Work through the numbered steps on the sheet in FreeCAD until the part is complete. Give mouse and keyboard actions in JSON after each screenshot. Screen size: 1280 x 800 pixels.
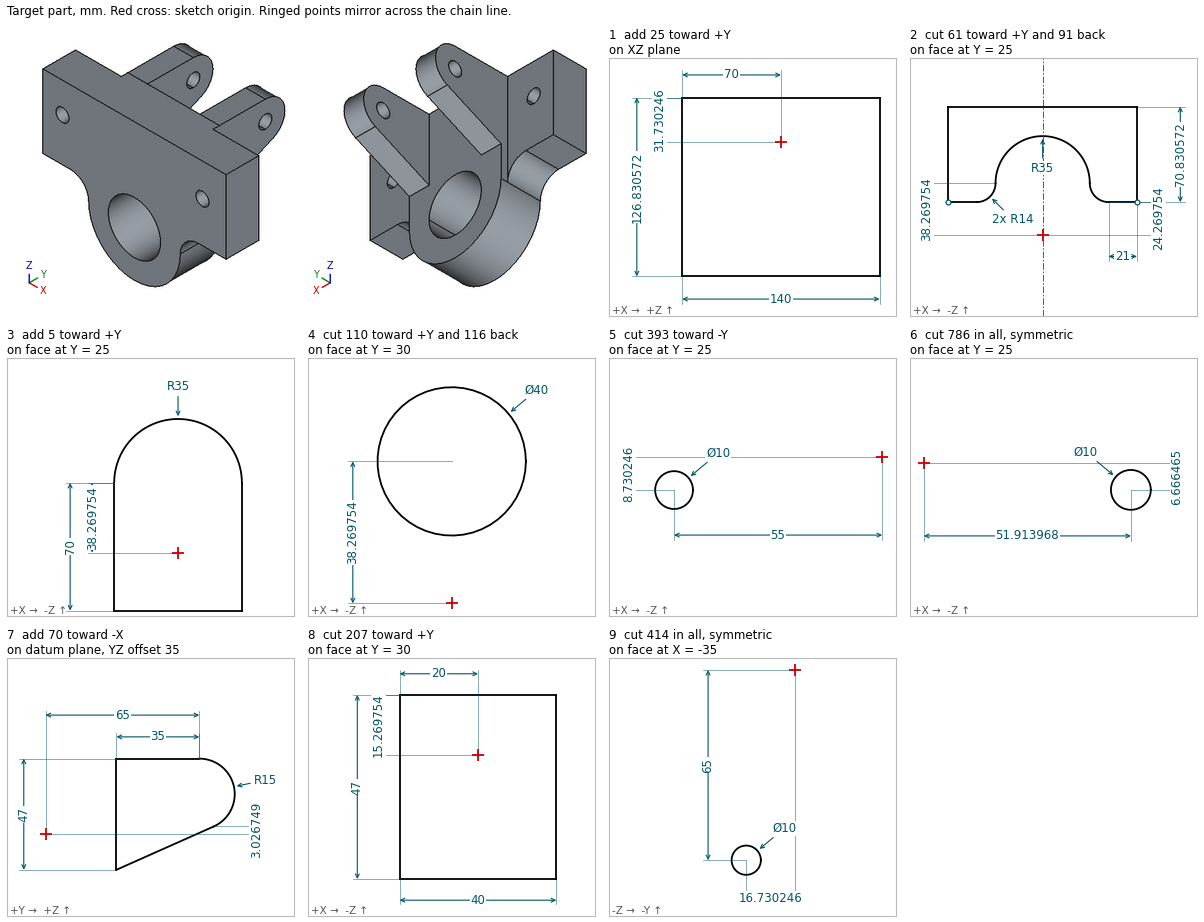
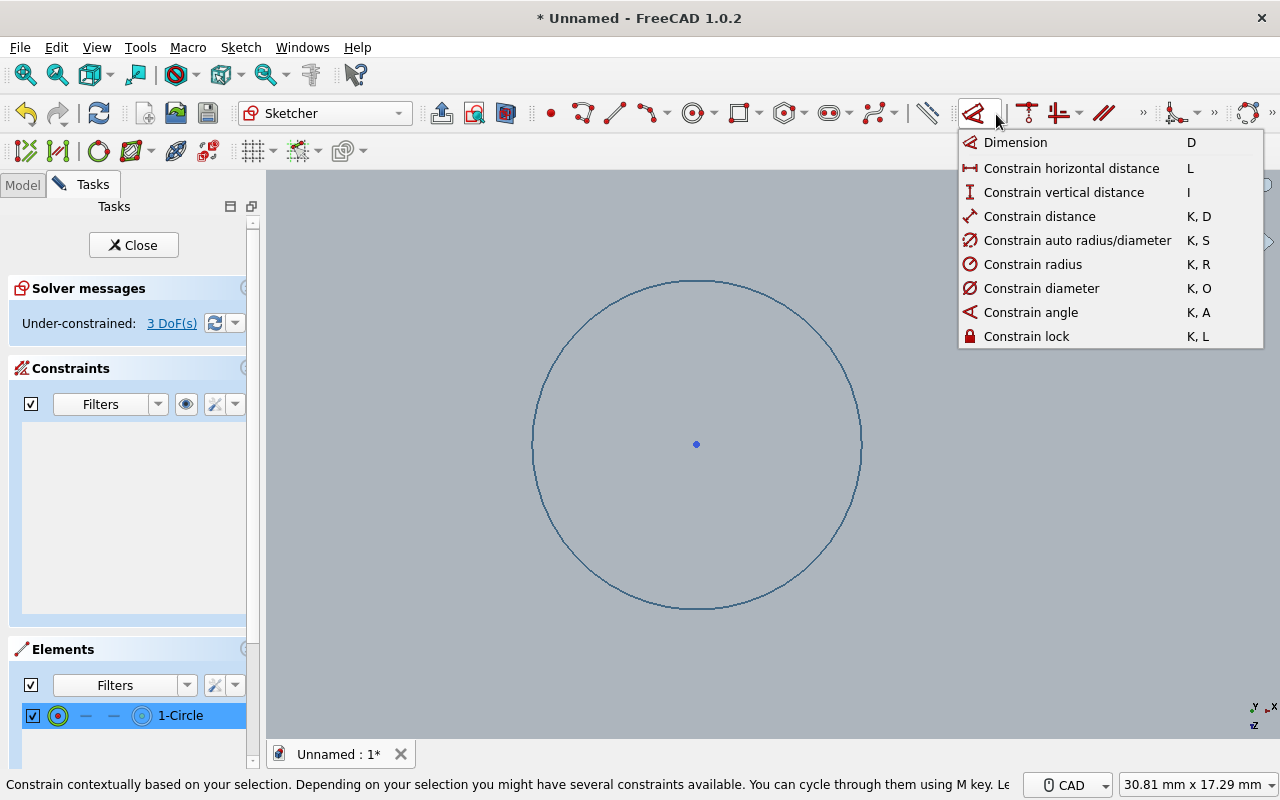
{"action": "left_click", "coordinate": [1111, 288]}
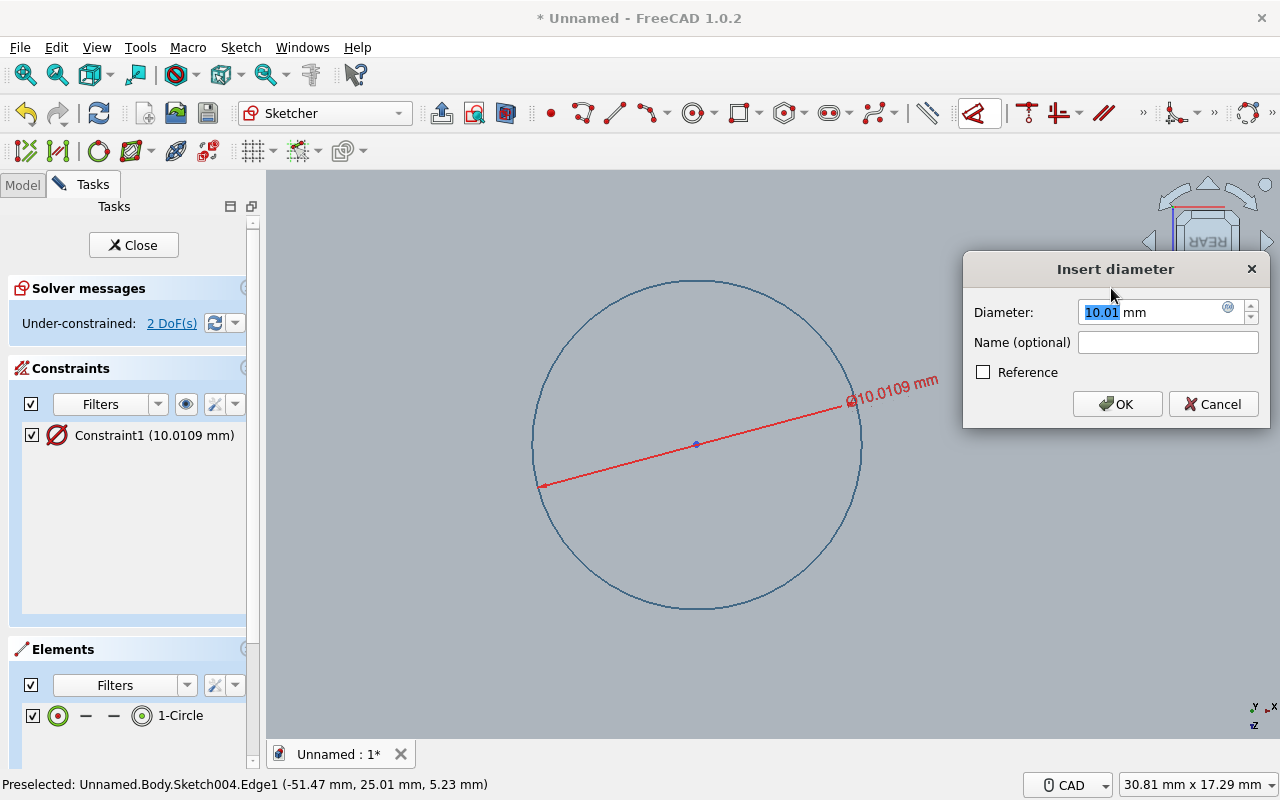
{"action": "type", "text": "10"}
{"action": "key", "text": "Return"}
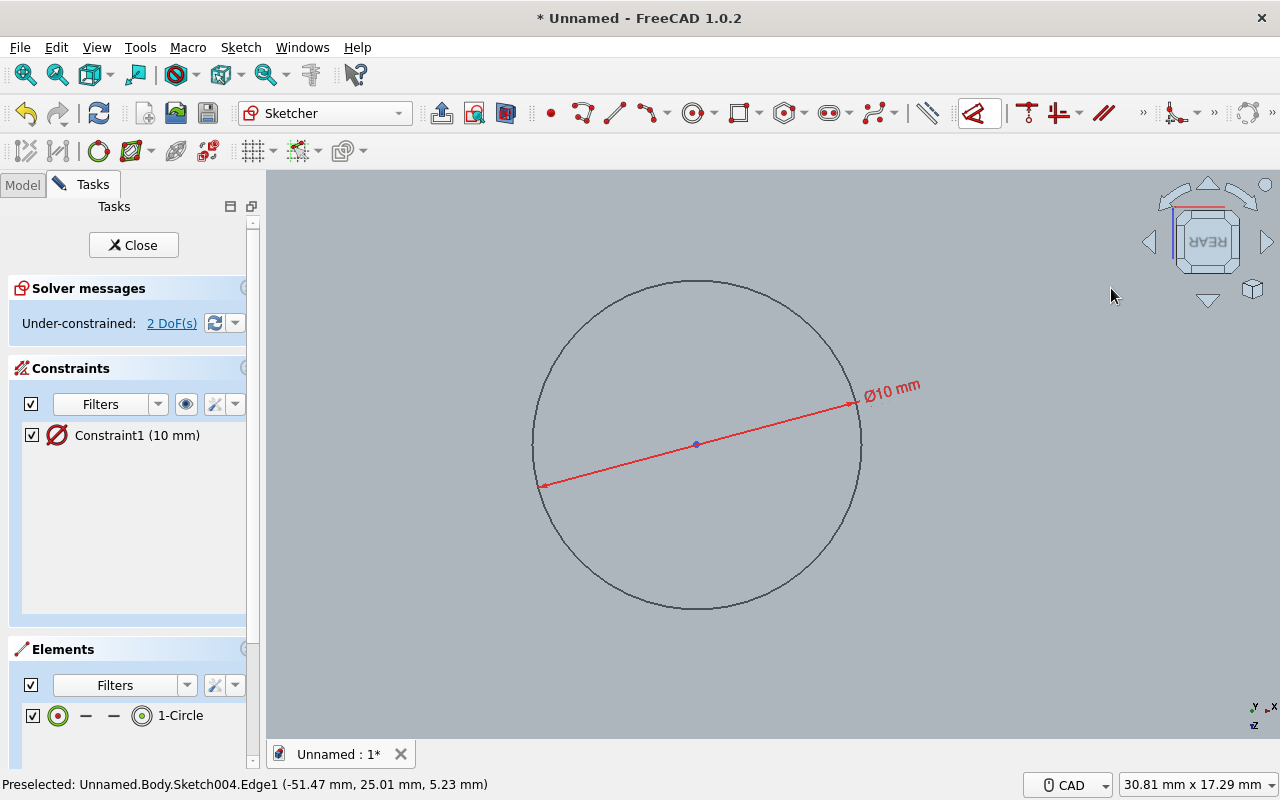
{"action": "left_click", "coordinate": [697, 445]}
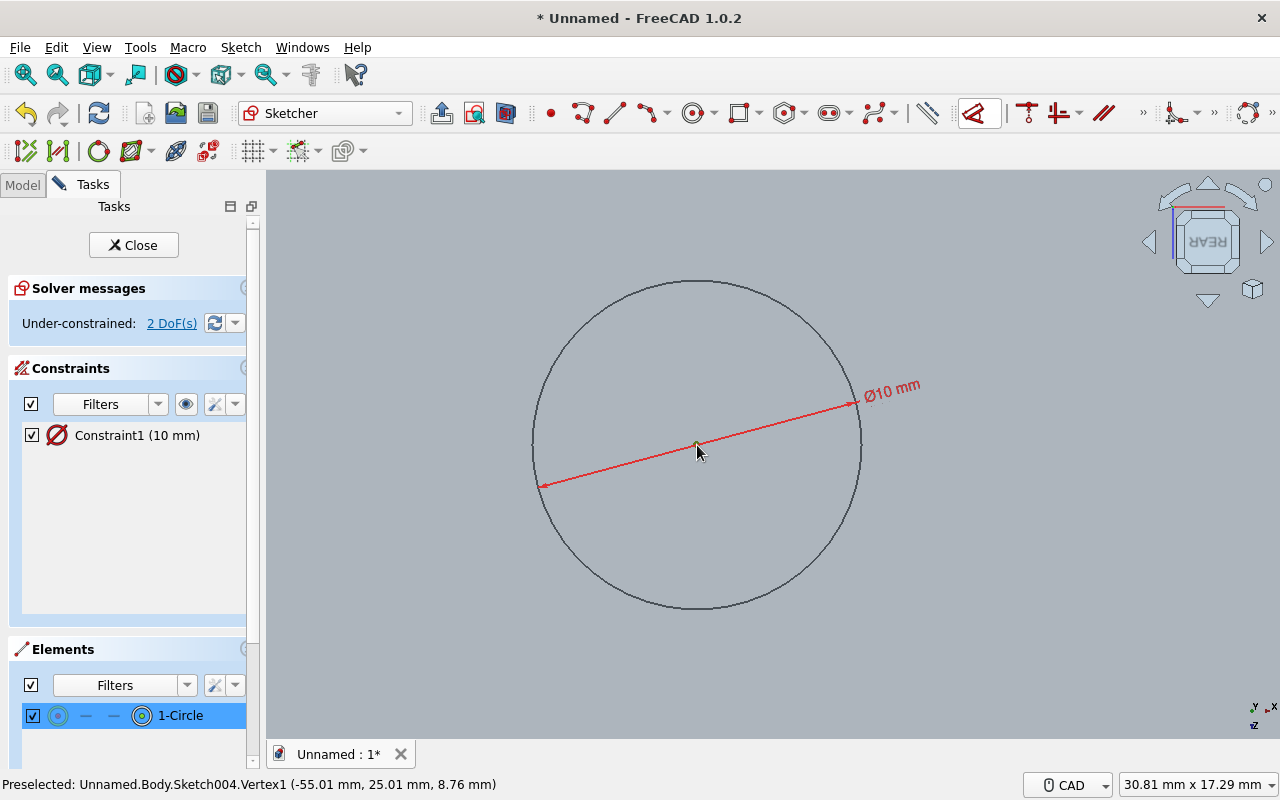
{"action": "key", "text": "l"}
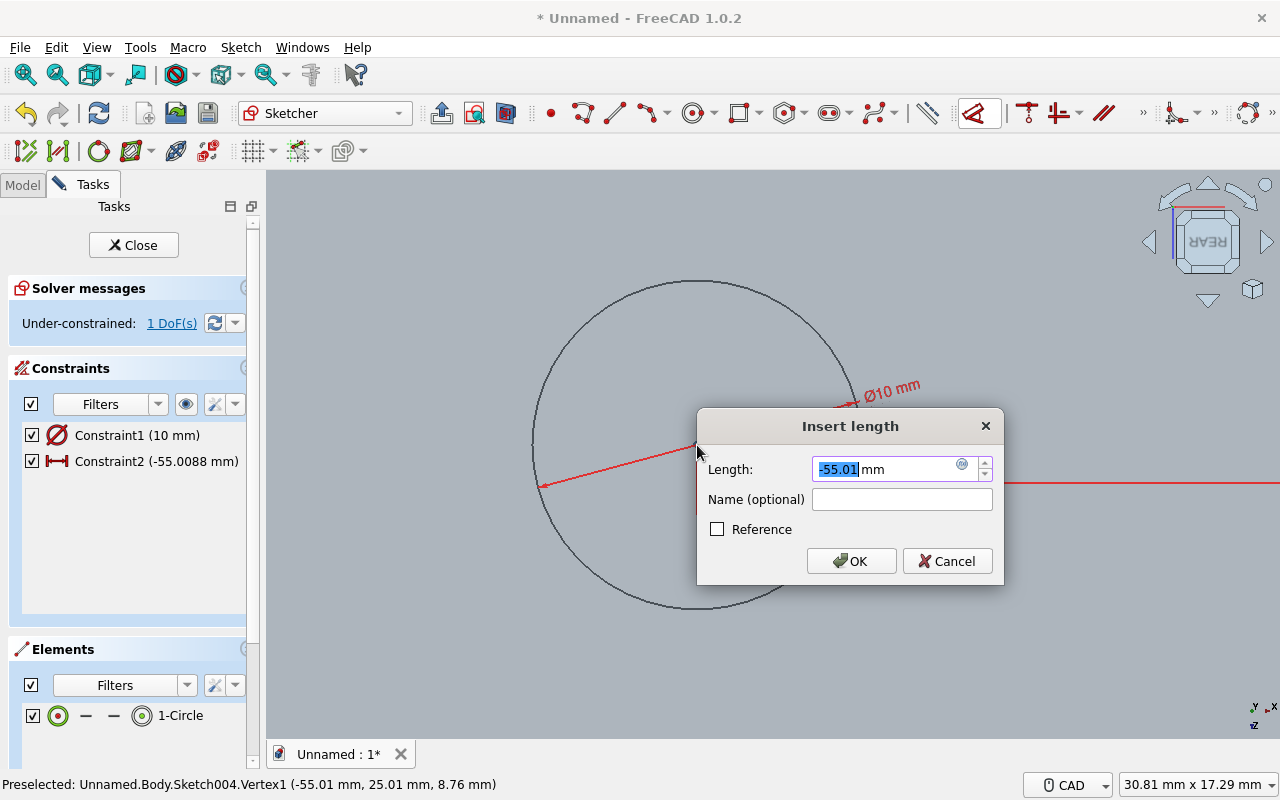
{"action": "type", "text": "-55"}
{"action": "key", "text": "Return"}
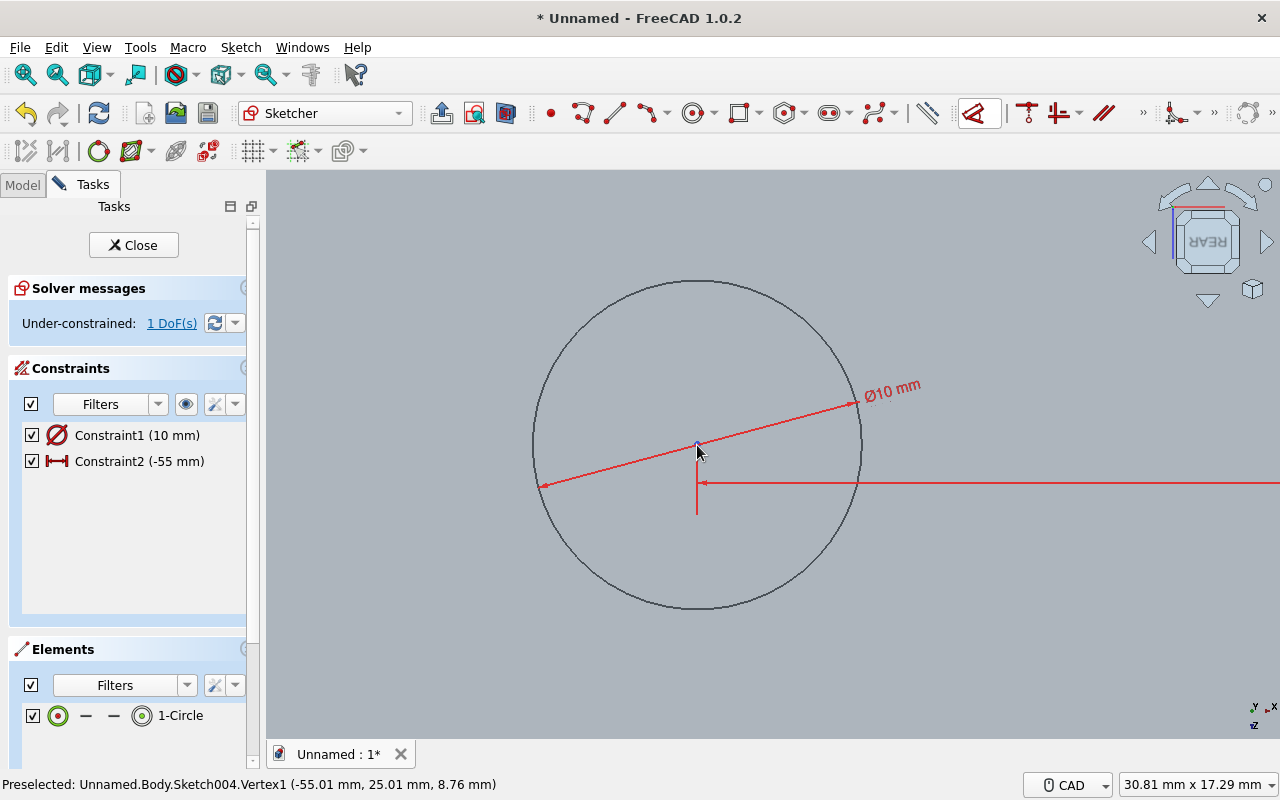
{"action": "left_click", "coordinate": [697, 445]}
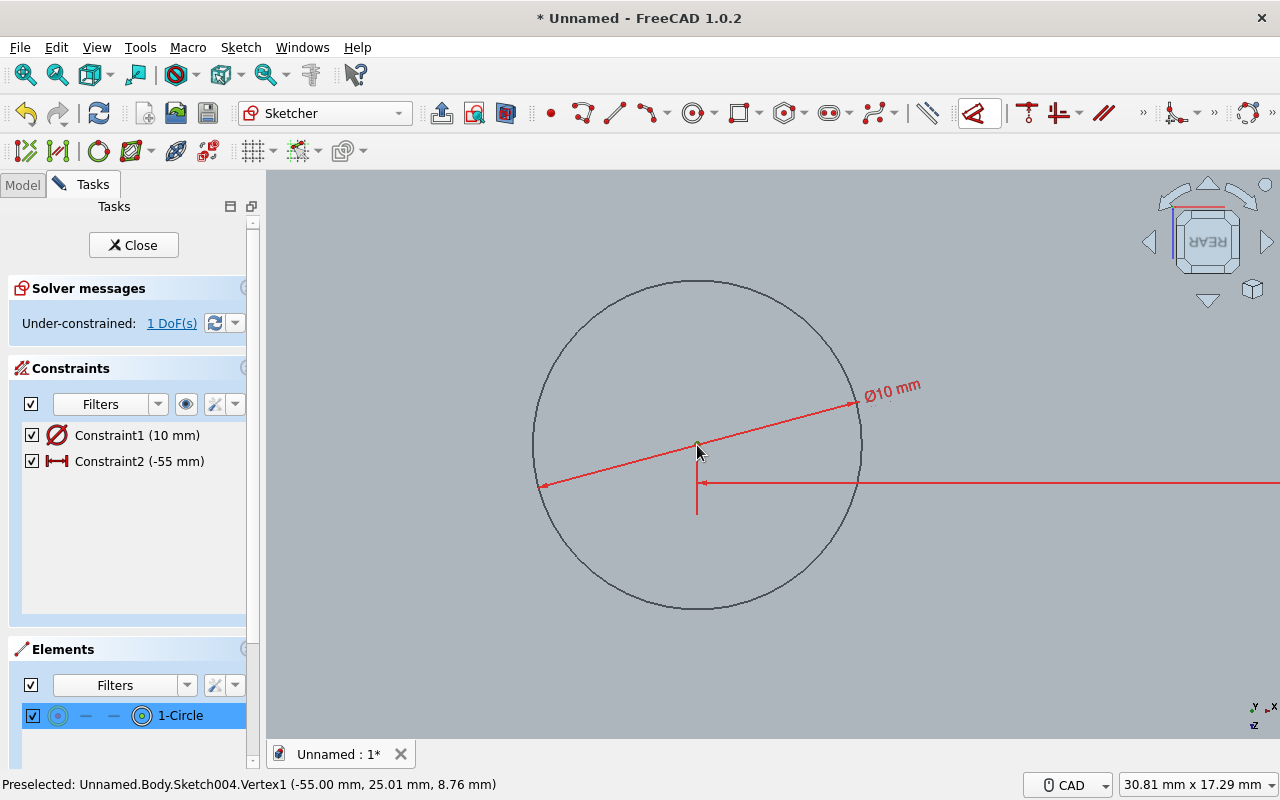
{"action": "key", "text": "i"}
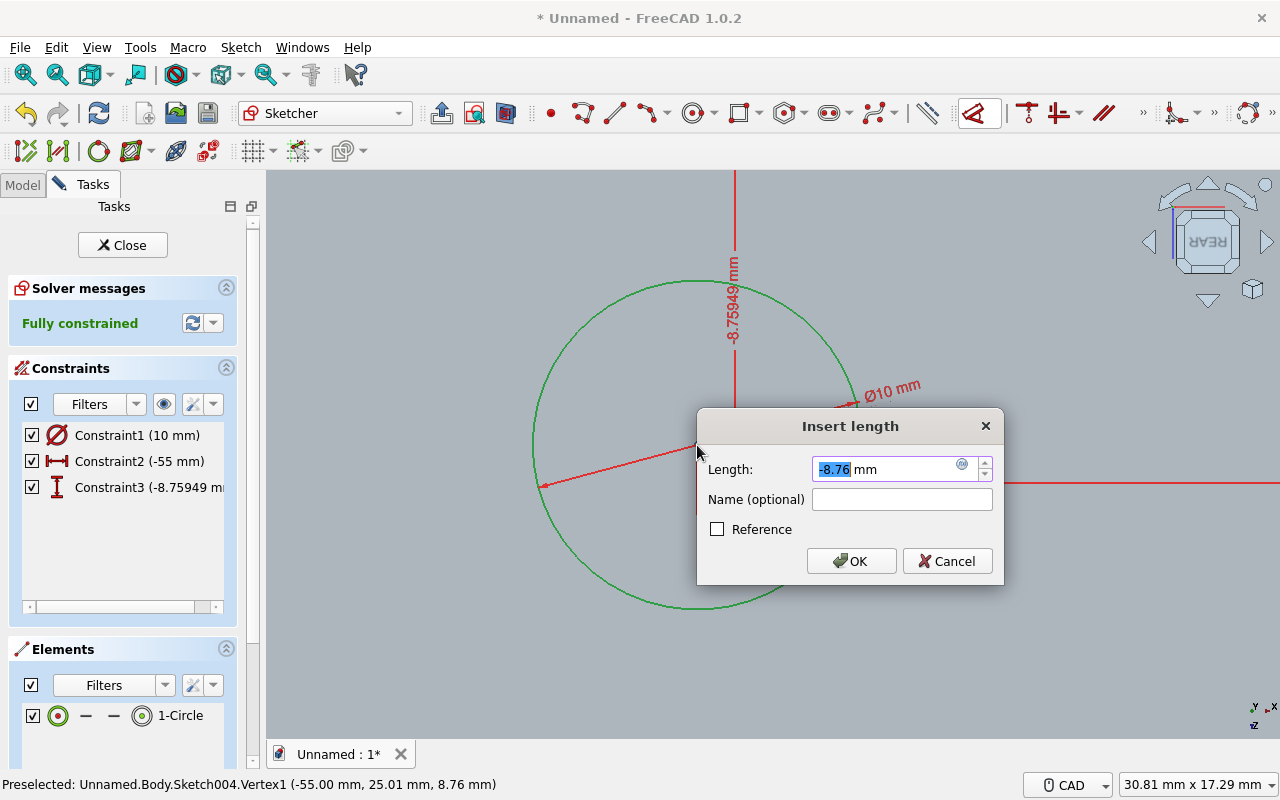
{"action": "type", "text": "-8.730246"}
{"action": "key", "text": "Return"}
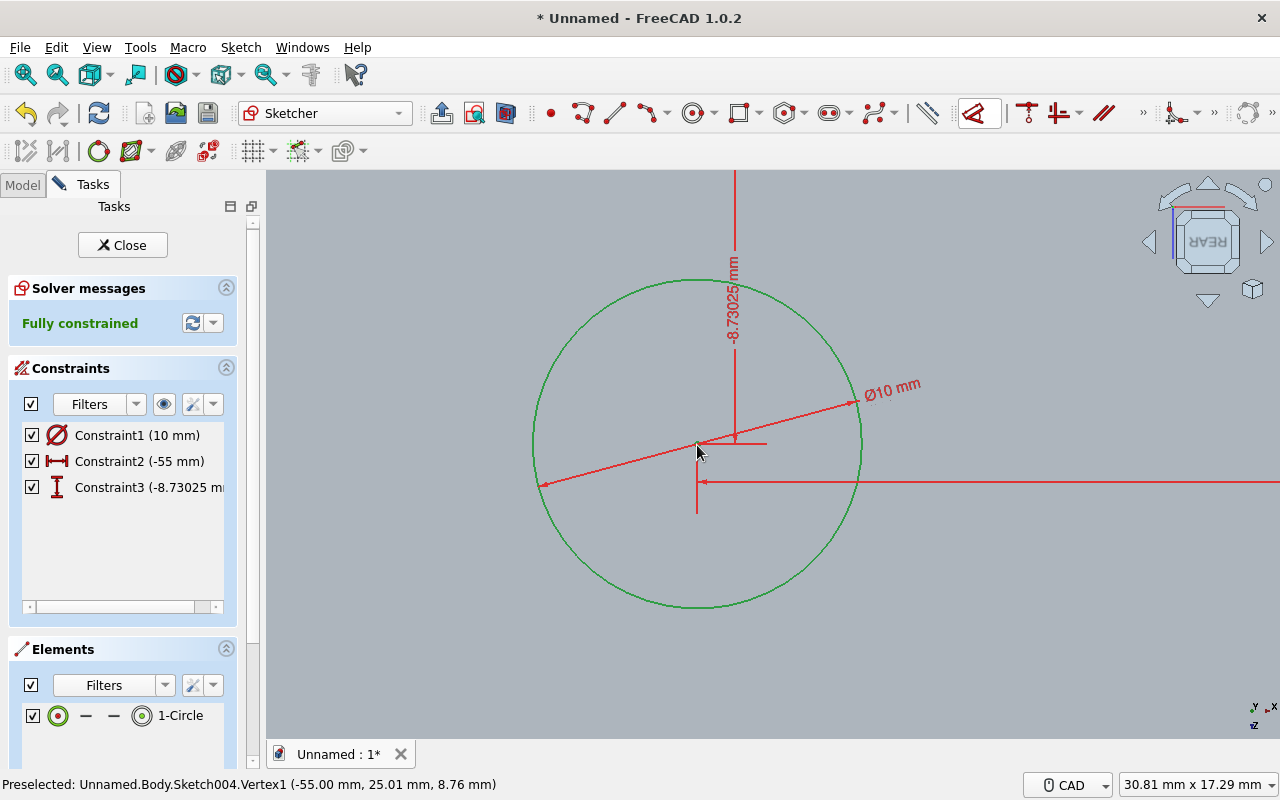
{"action": "left_click", "coordinate": [123, 245]}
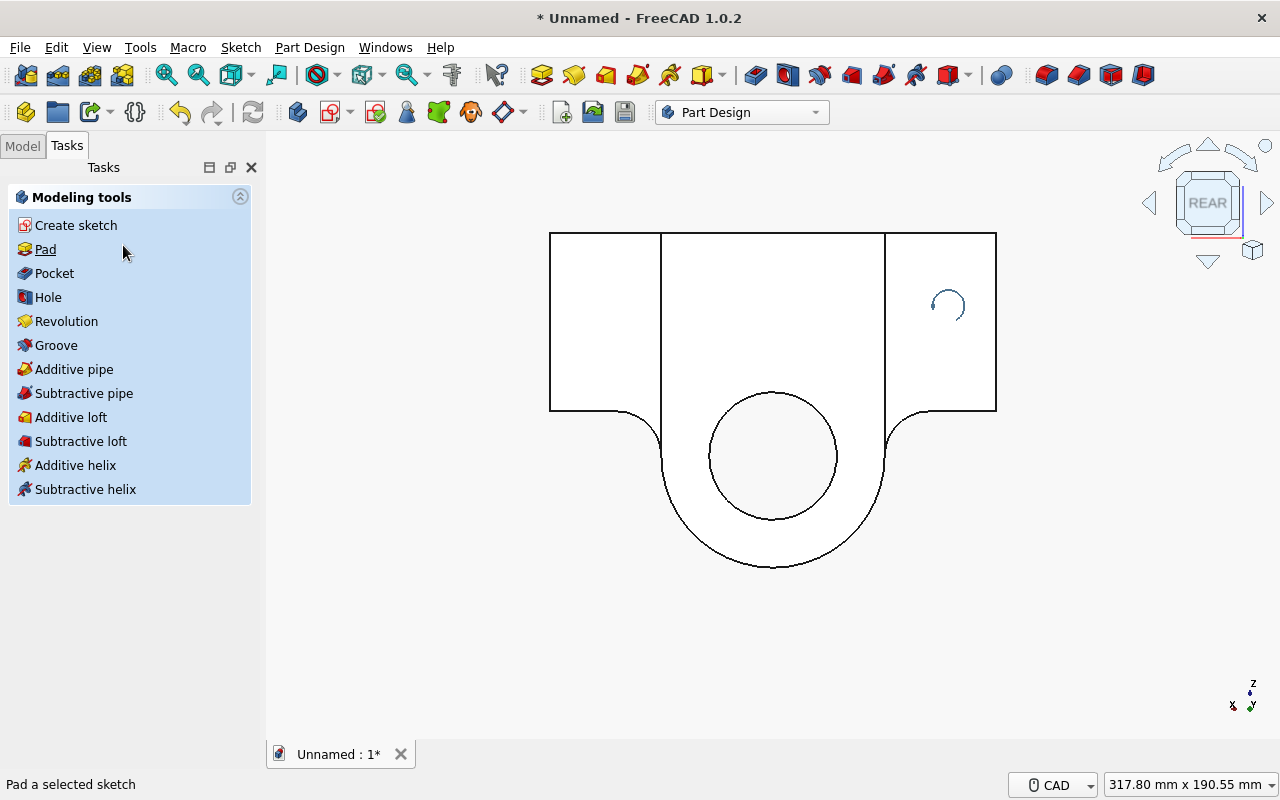
{"action": "left_click", "coordinate": [756, 76]}